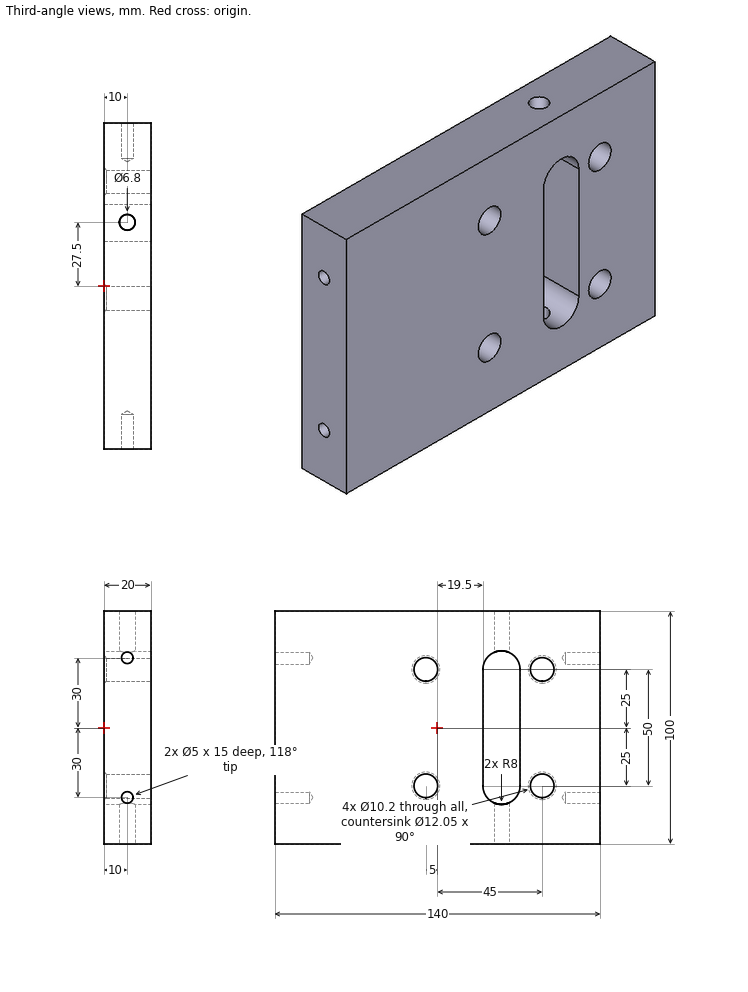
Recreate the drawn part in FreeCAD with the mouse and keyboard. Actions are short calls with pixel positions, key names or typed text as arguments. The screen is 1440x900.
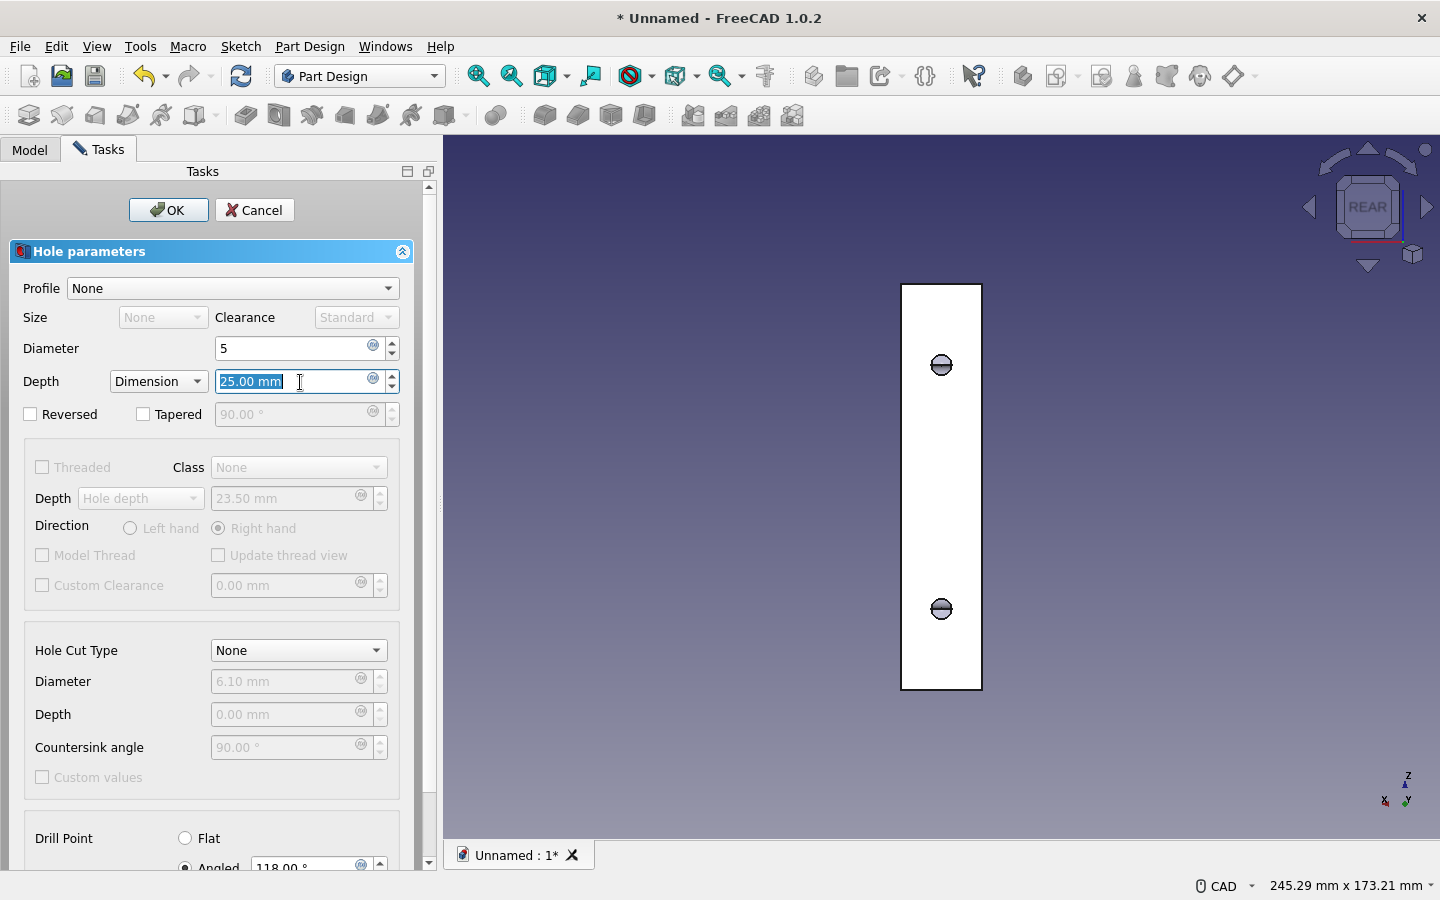
text(15)
key(Tab)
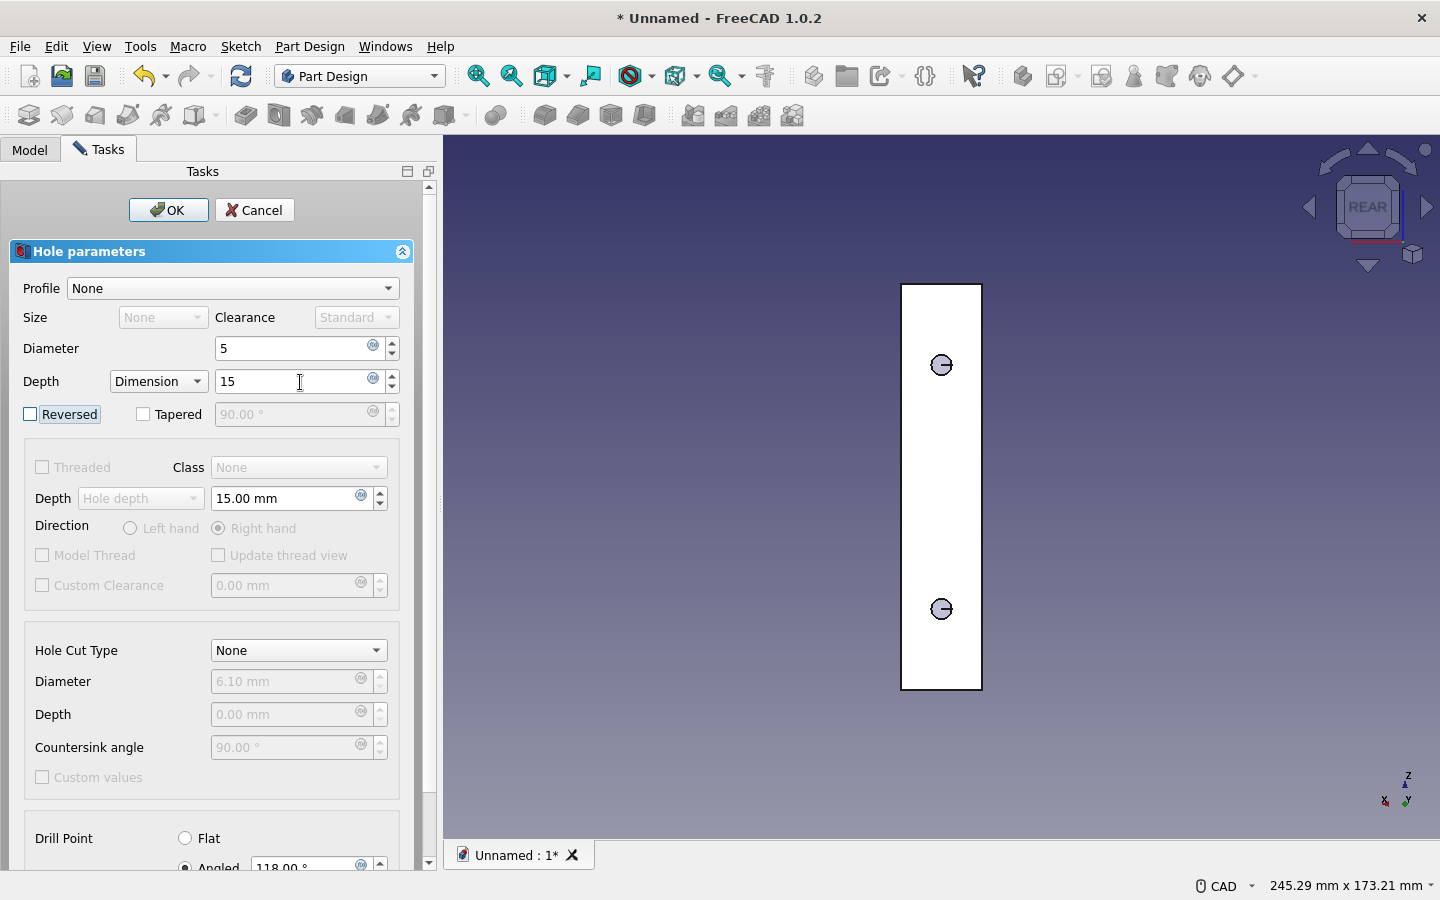
click(169, 210)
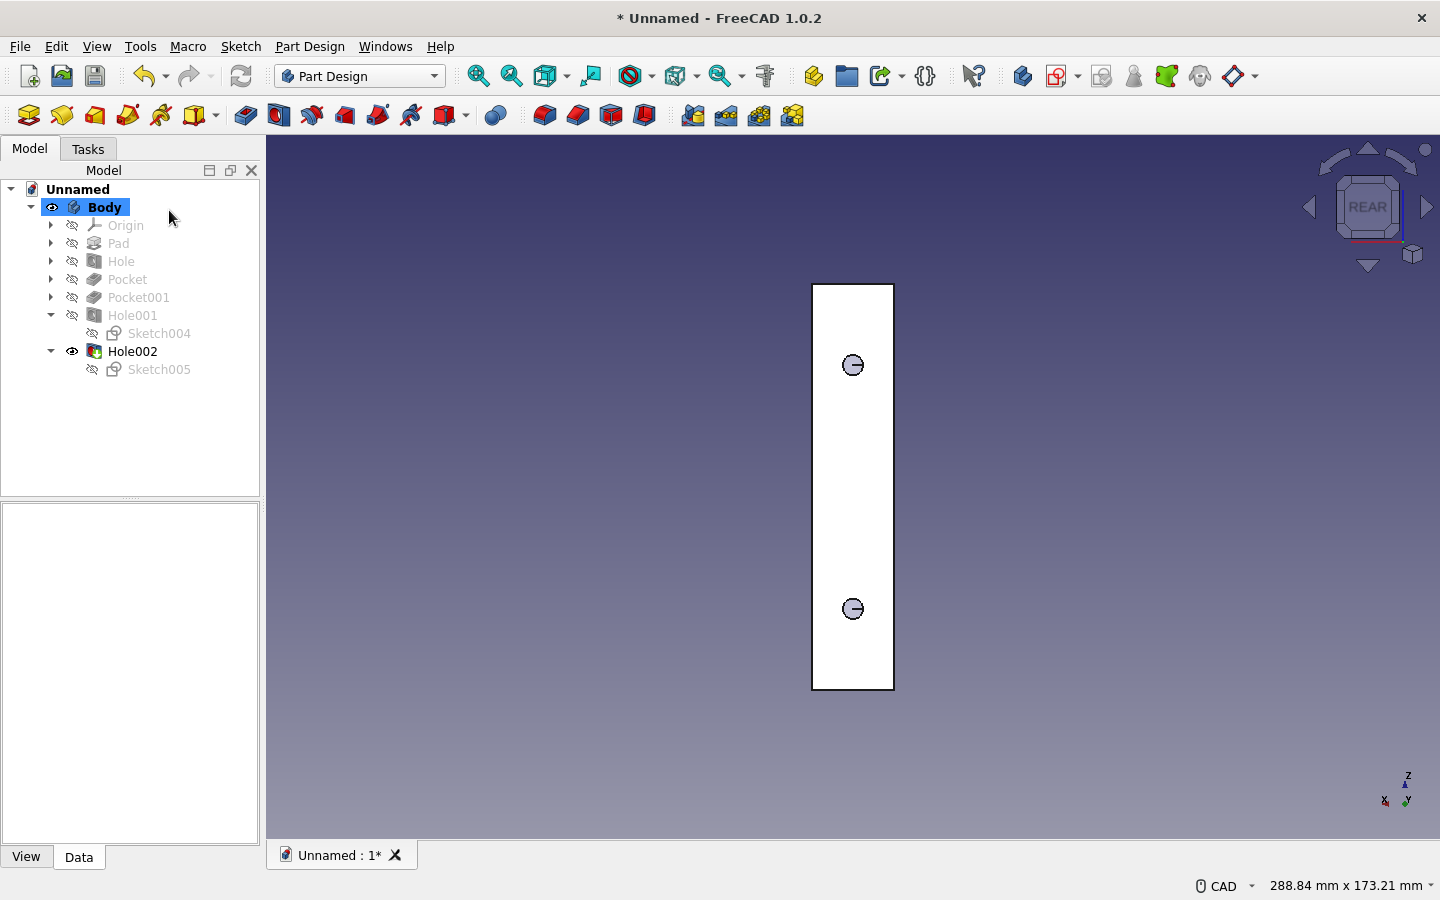
key(0)